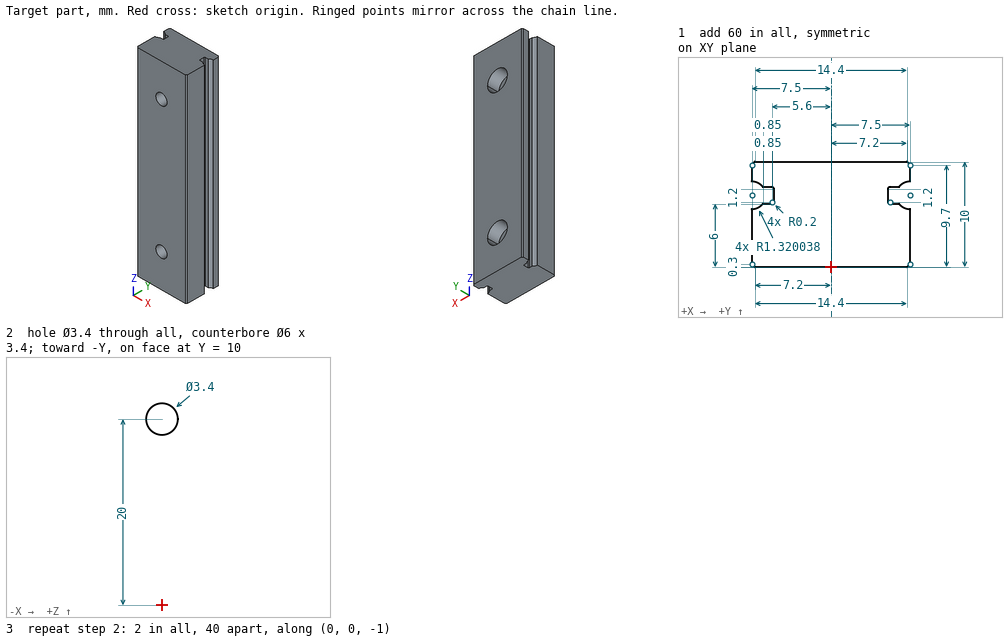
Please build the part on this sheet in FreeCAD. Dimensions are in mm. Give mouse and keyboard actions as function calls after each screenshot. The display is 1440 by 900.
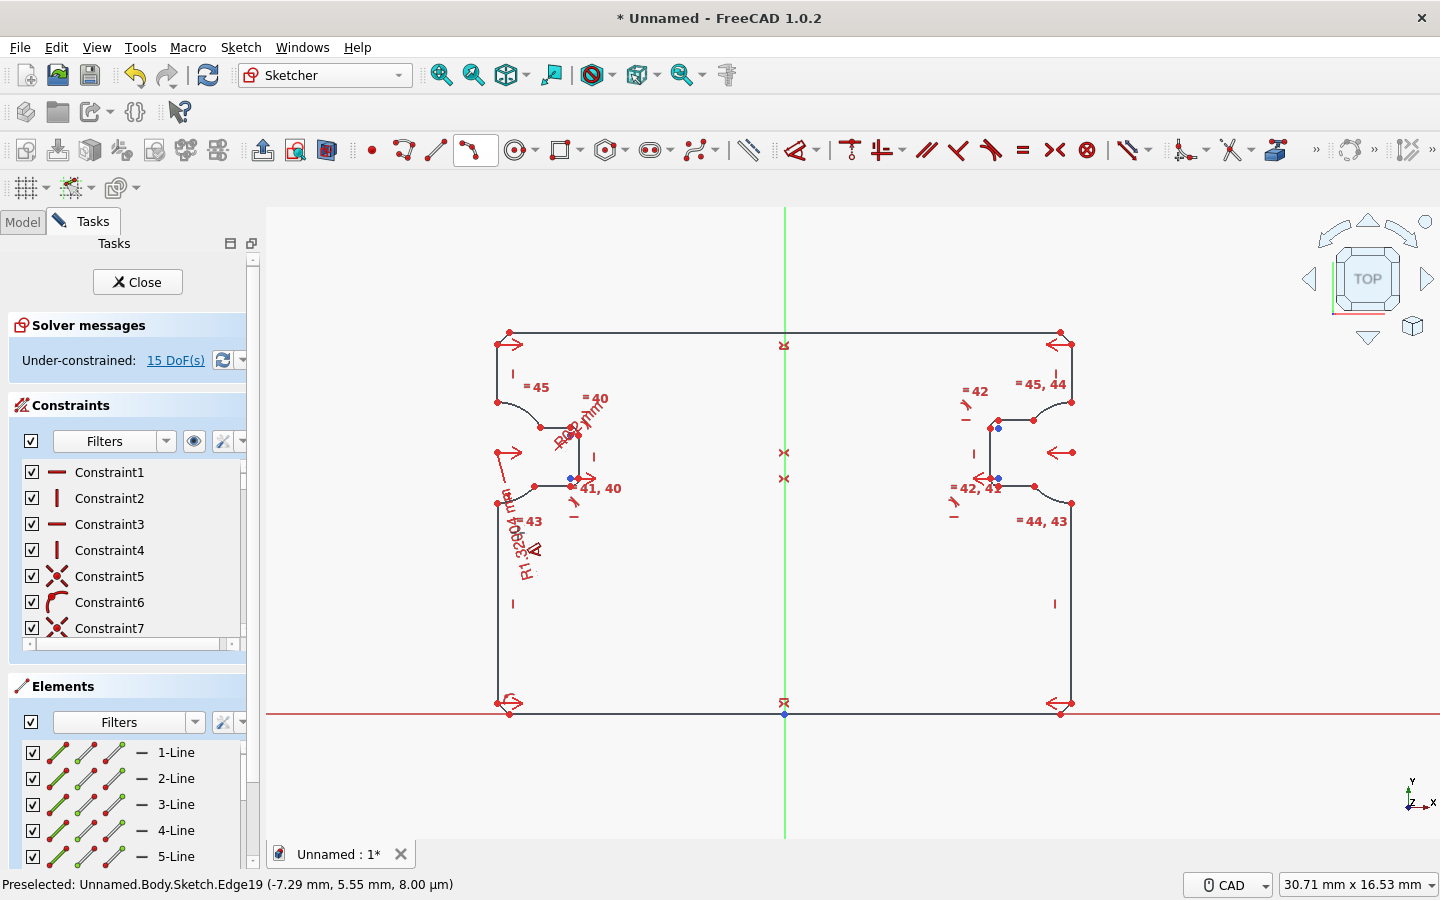
scroll(571, 486, up, 3)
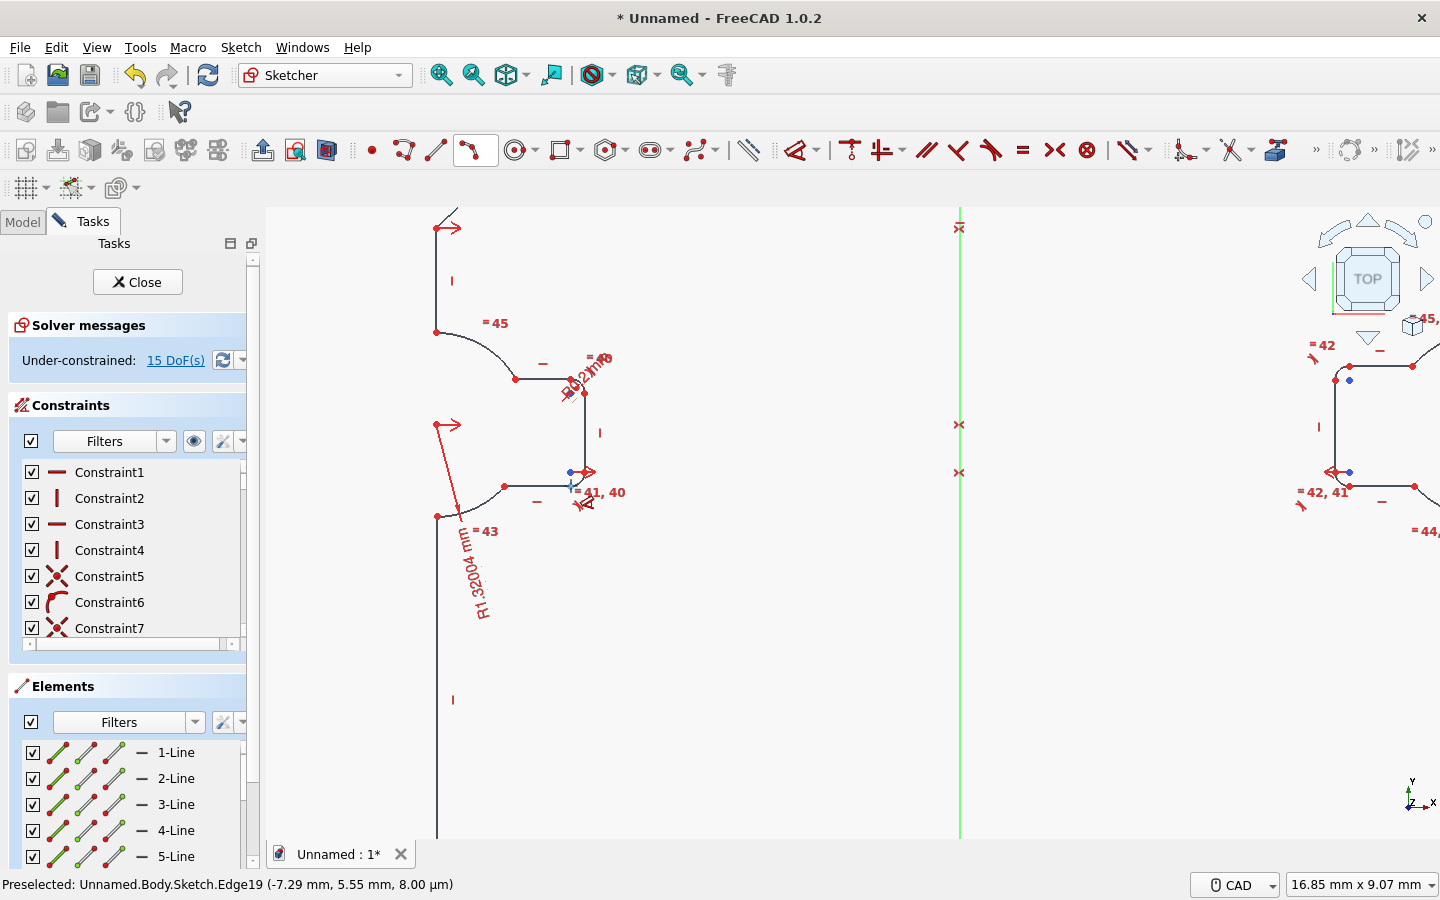
click(571, 486)
click(537, 649)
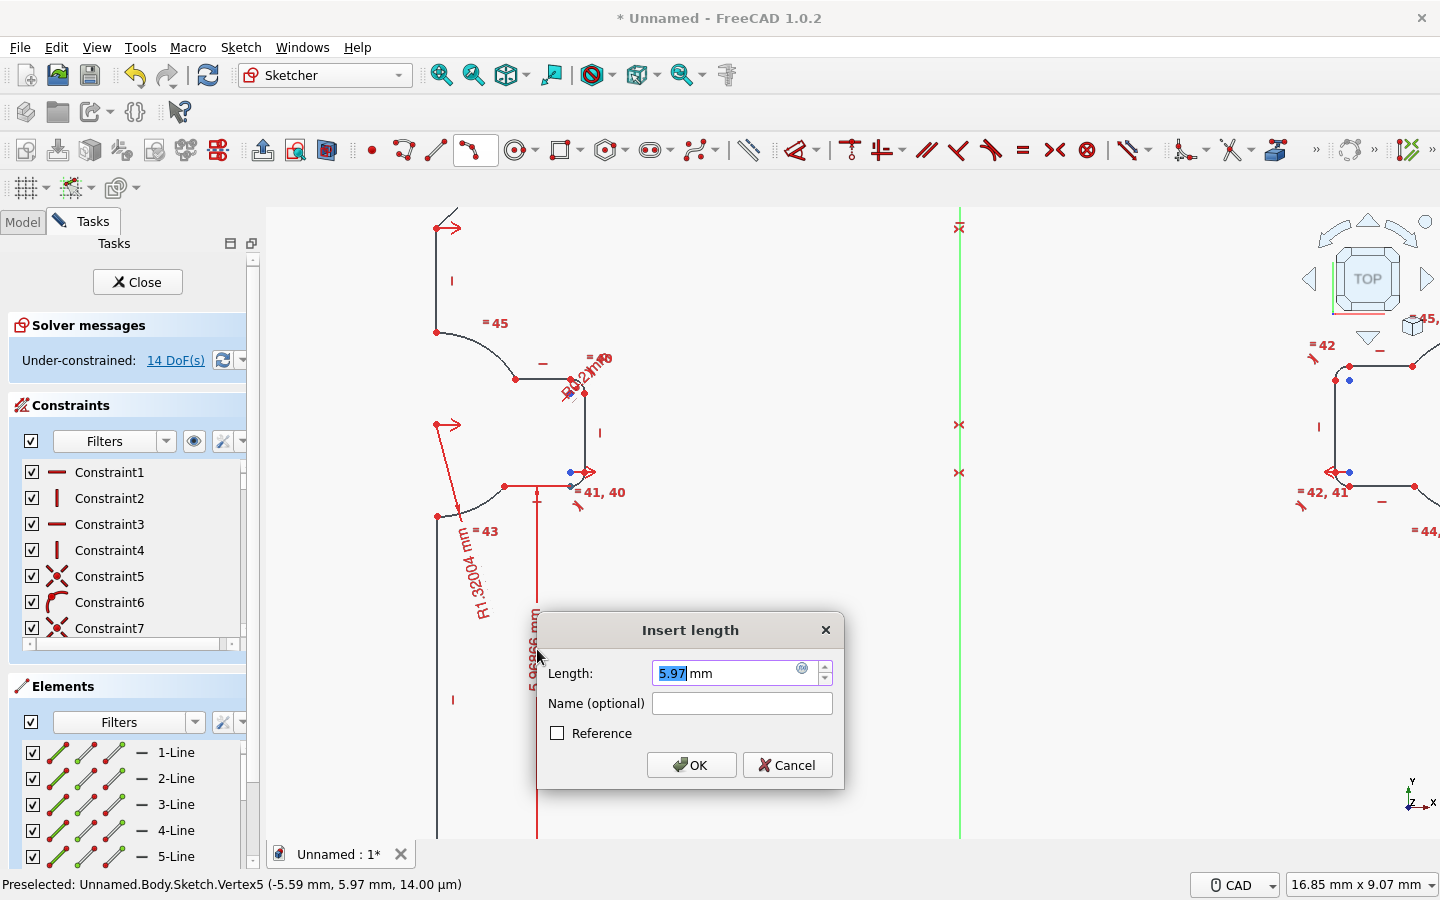
text(6)
key(Return)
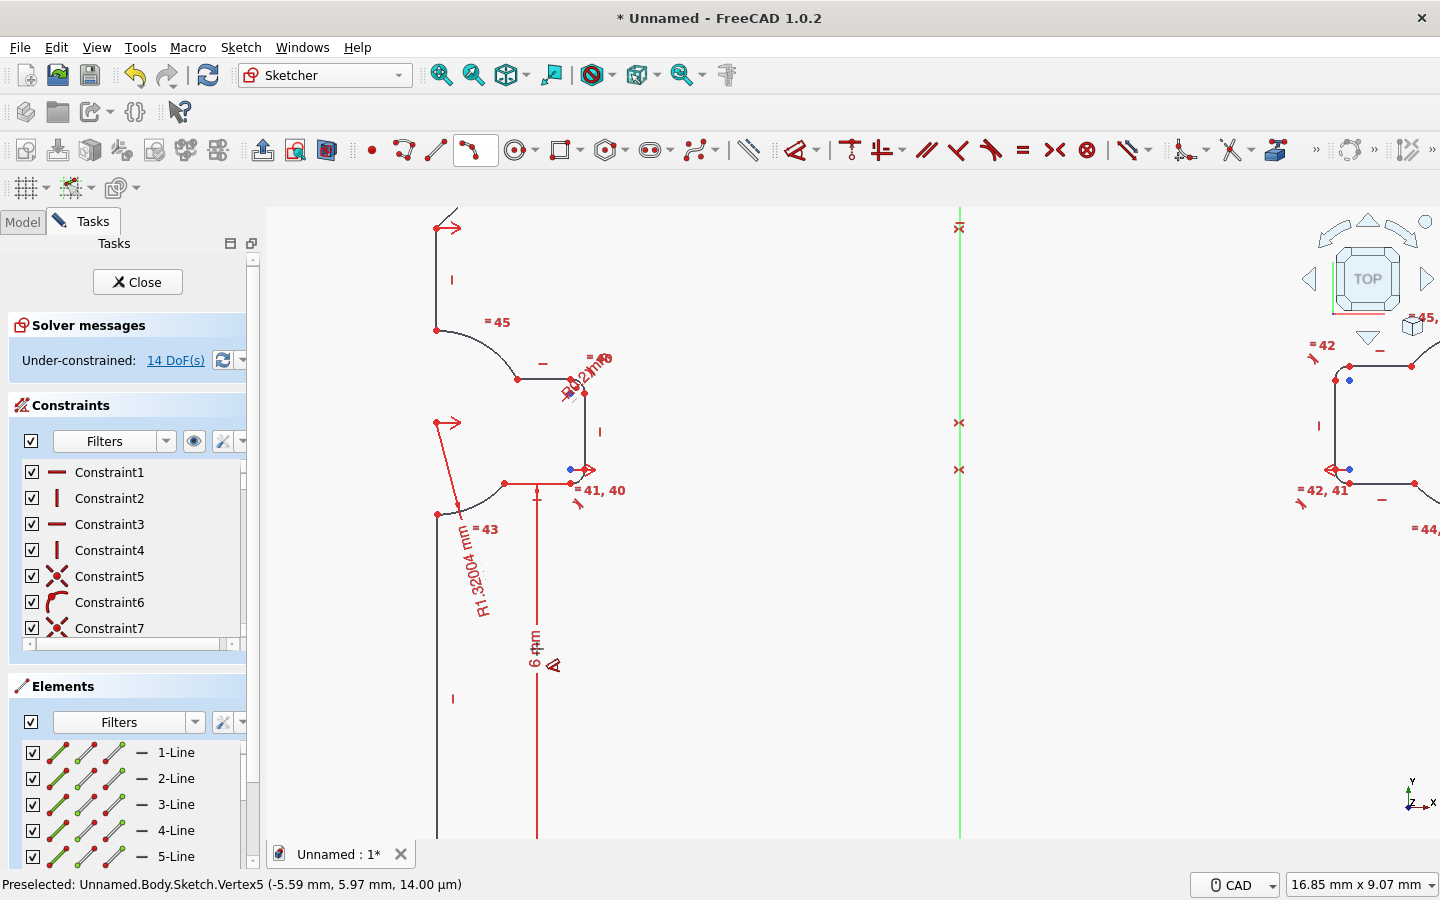
click(585, 416)
click(551, 432)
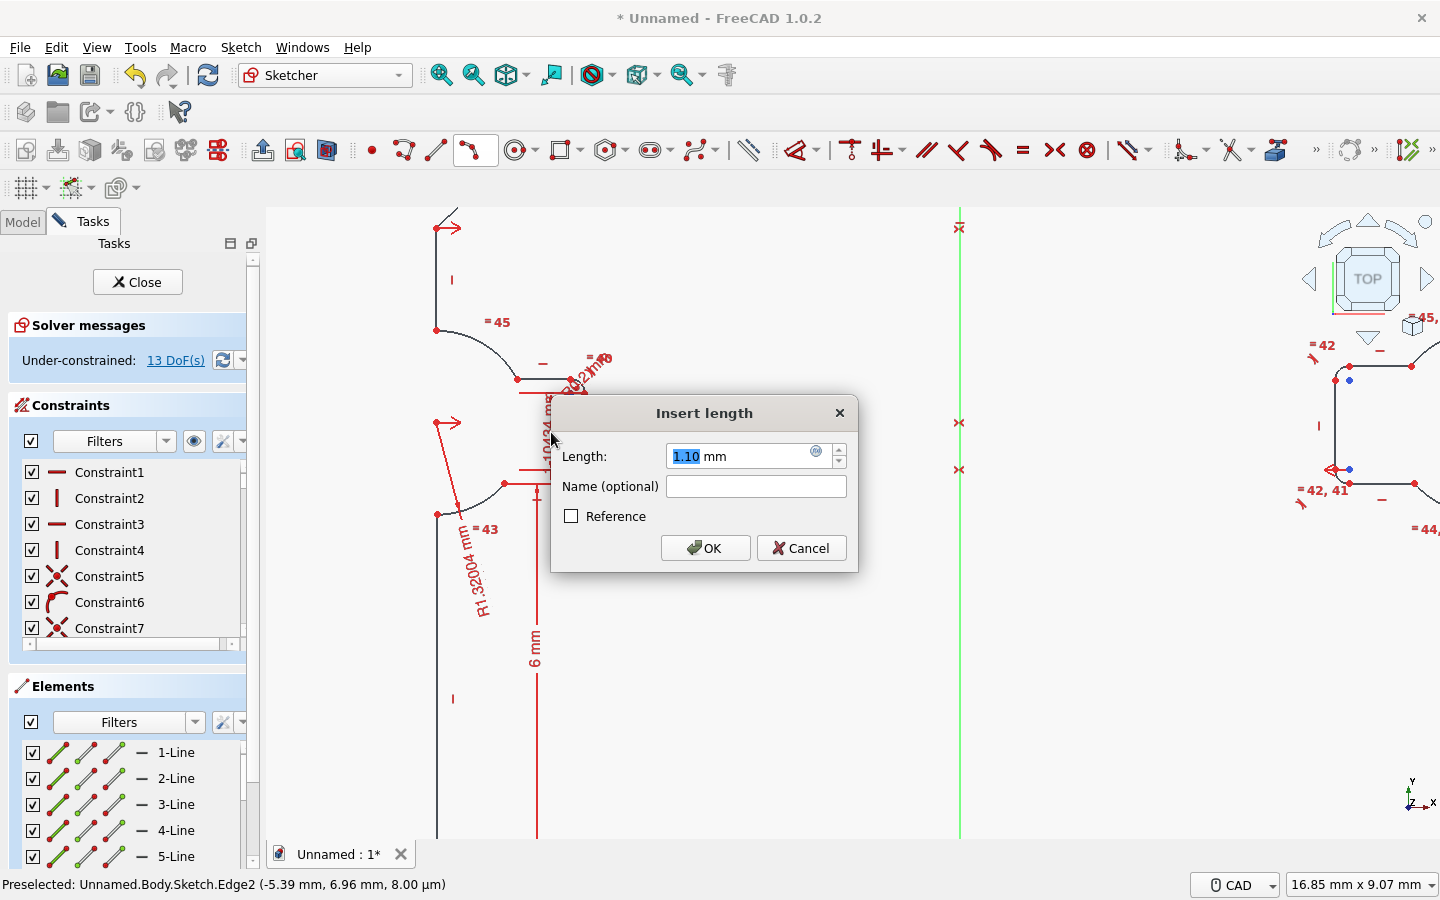
text(1.2)
key(Return)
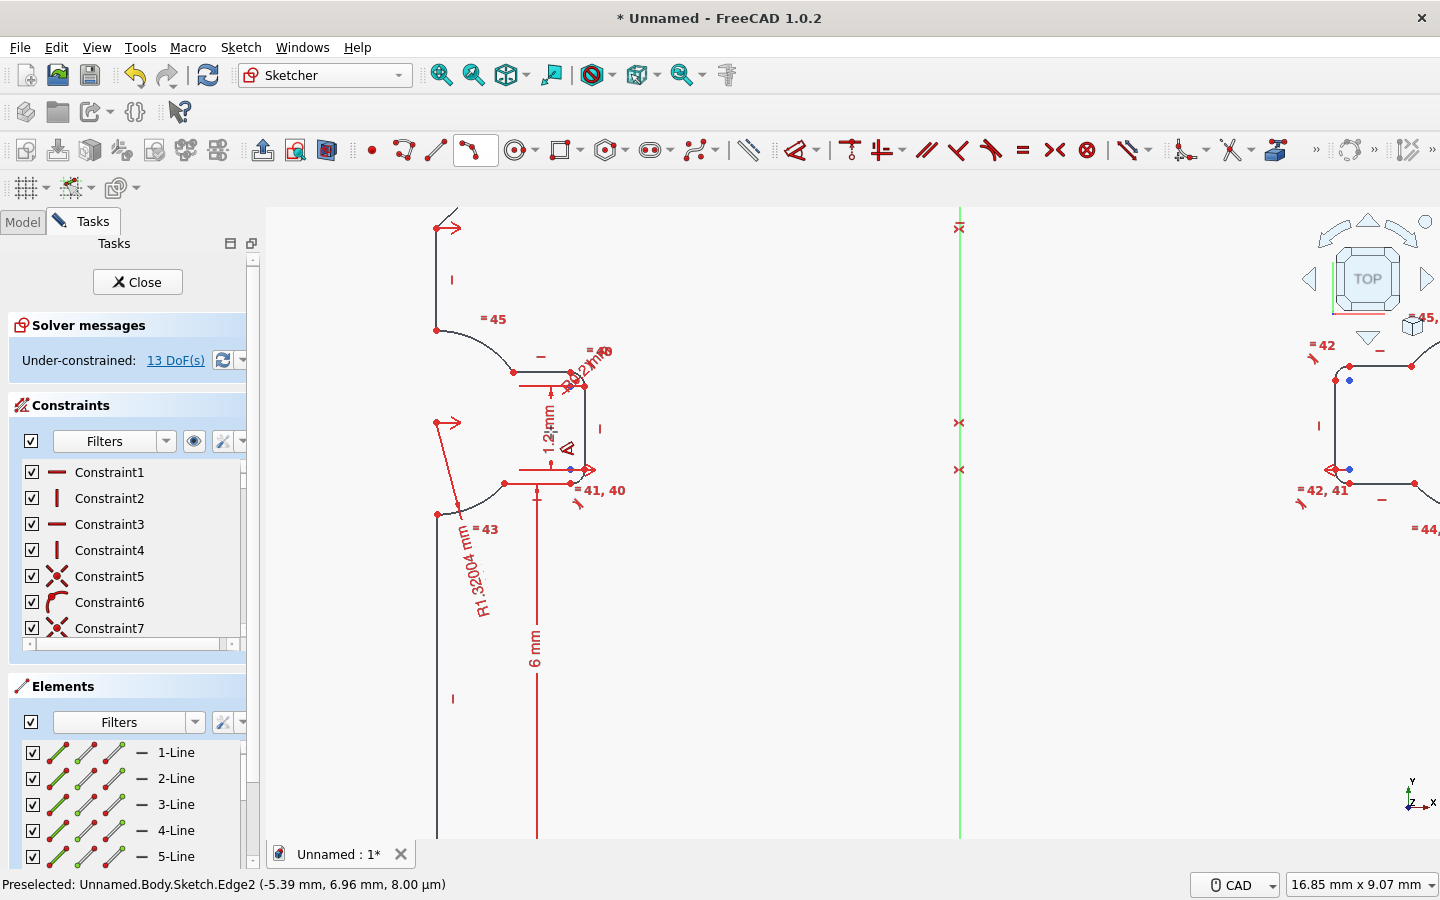
scroll(571, 486, down, 3)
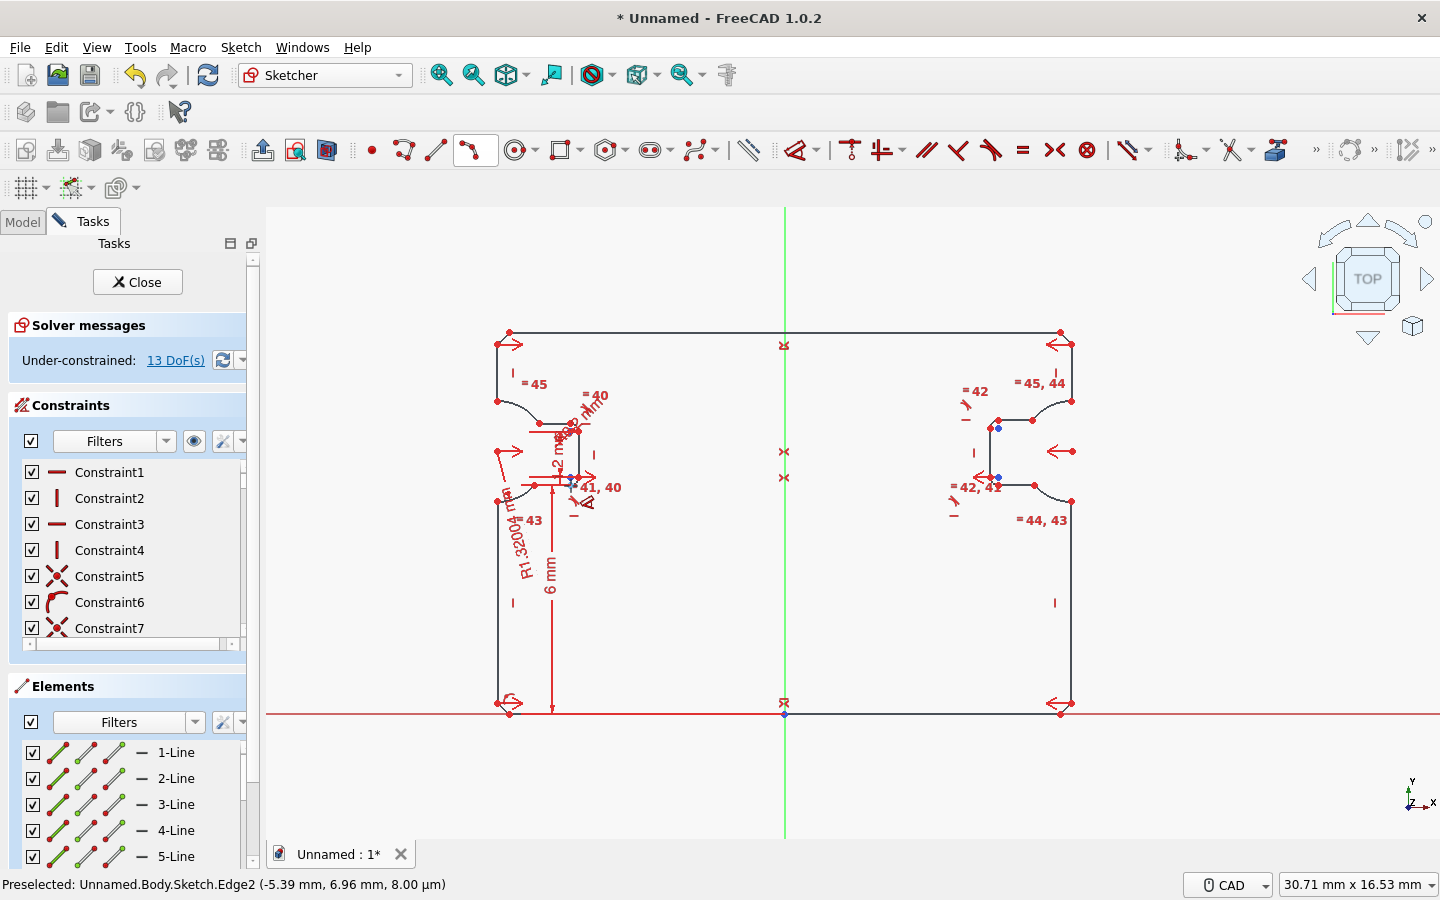
click(990, 463)
click(1024, 453)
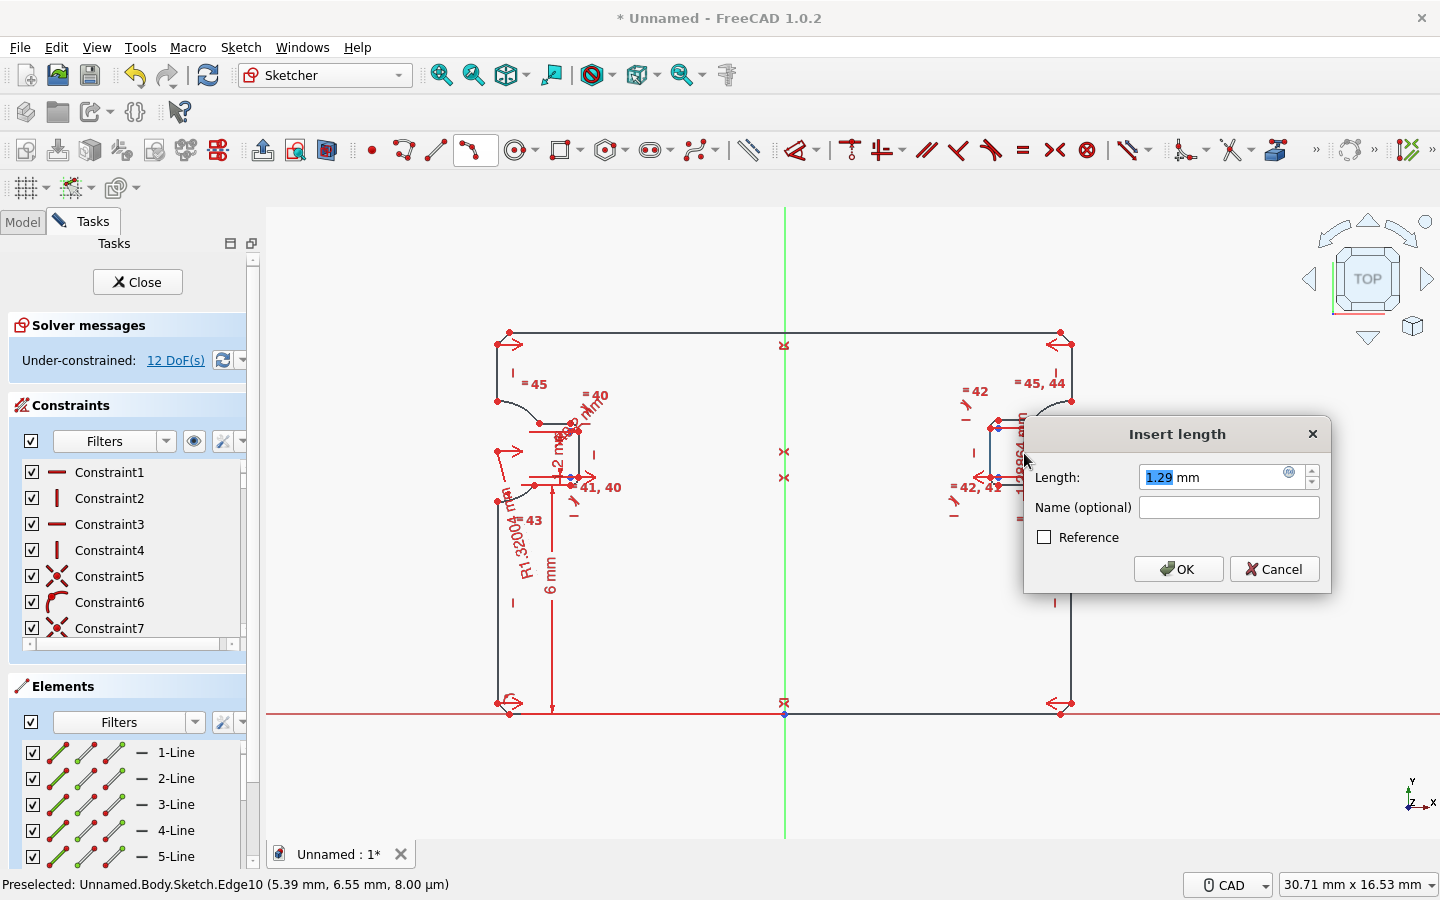
text(1.2)
key(Return)